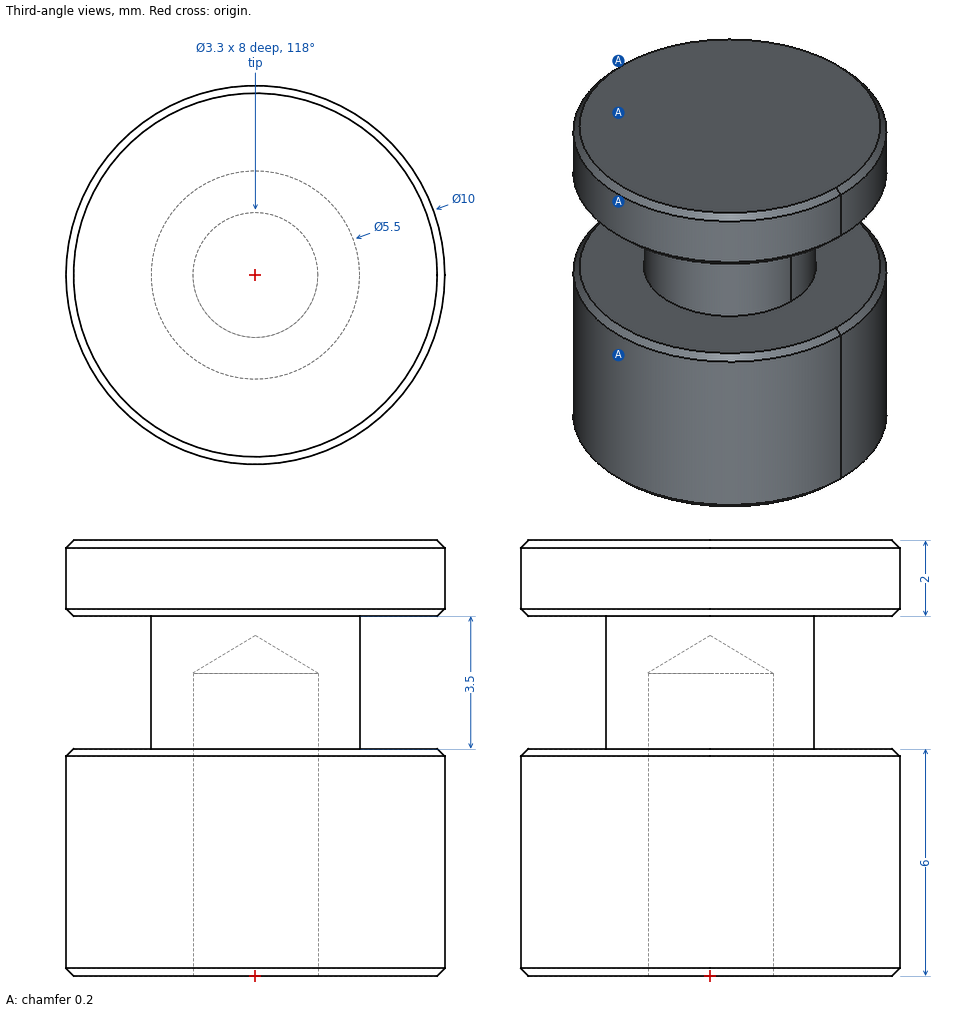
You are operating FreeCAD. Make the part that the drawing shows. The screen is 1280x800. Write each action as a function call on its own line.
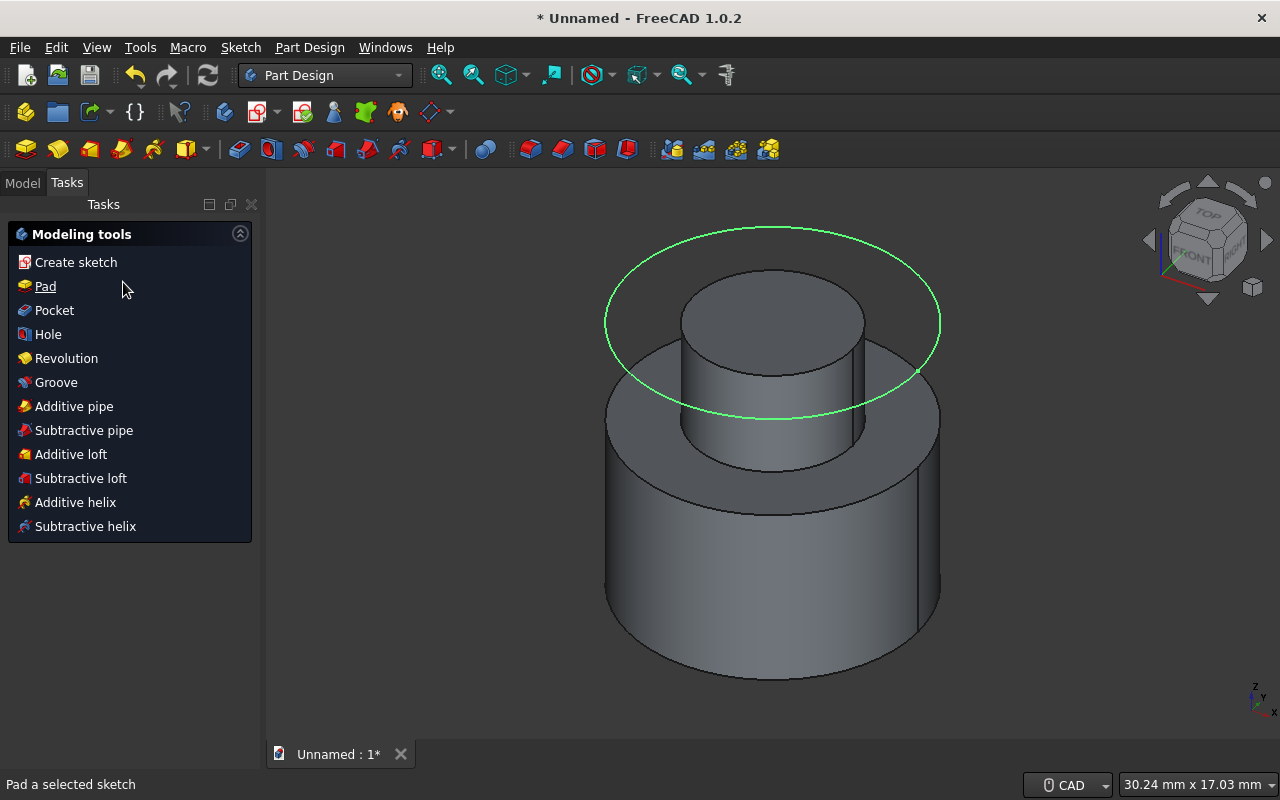
click(26, 150)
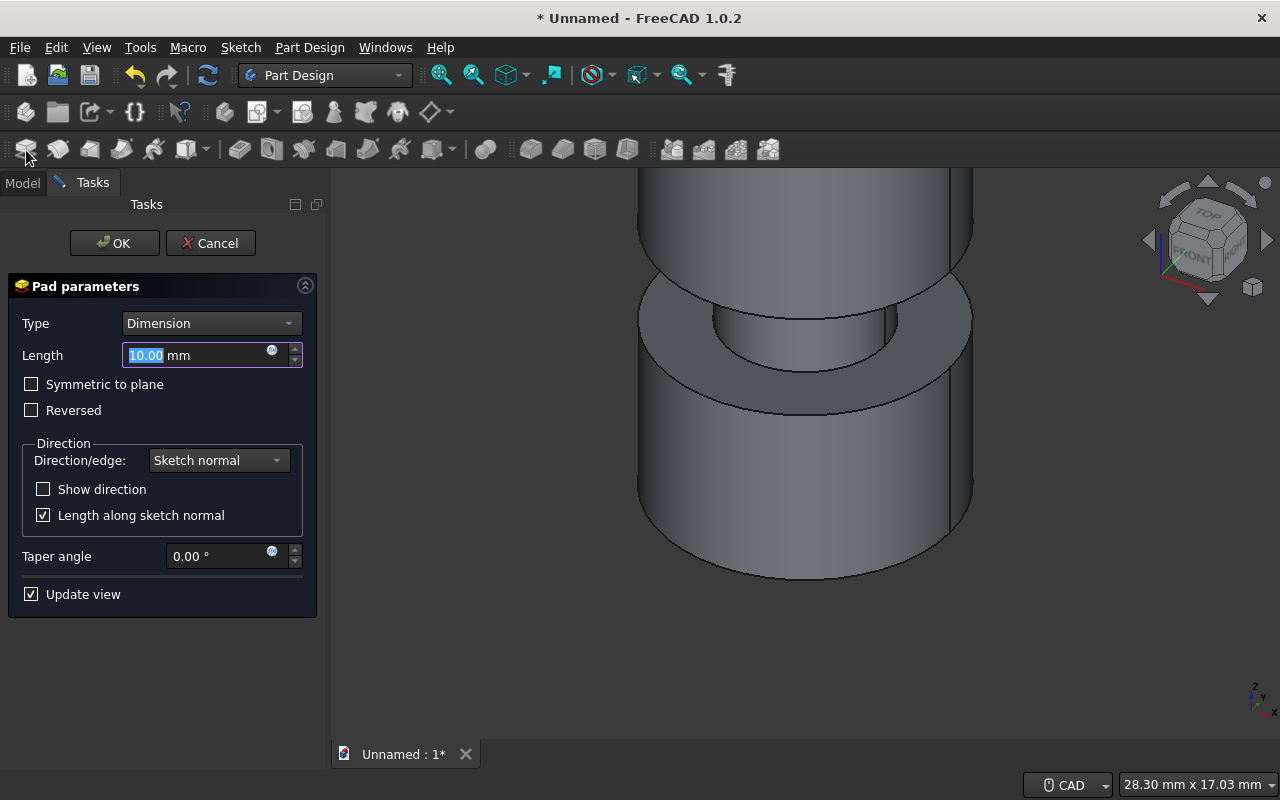
text(2)
key(Tab)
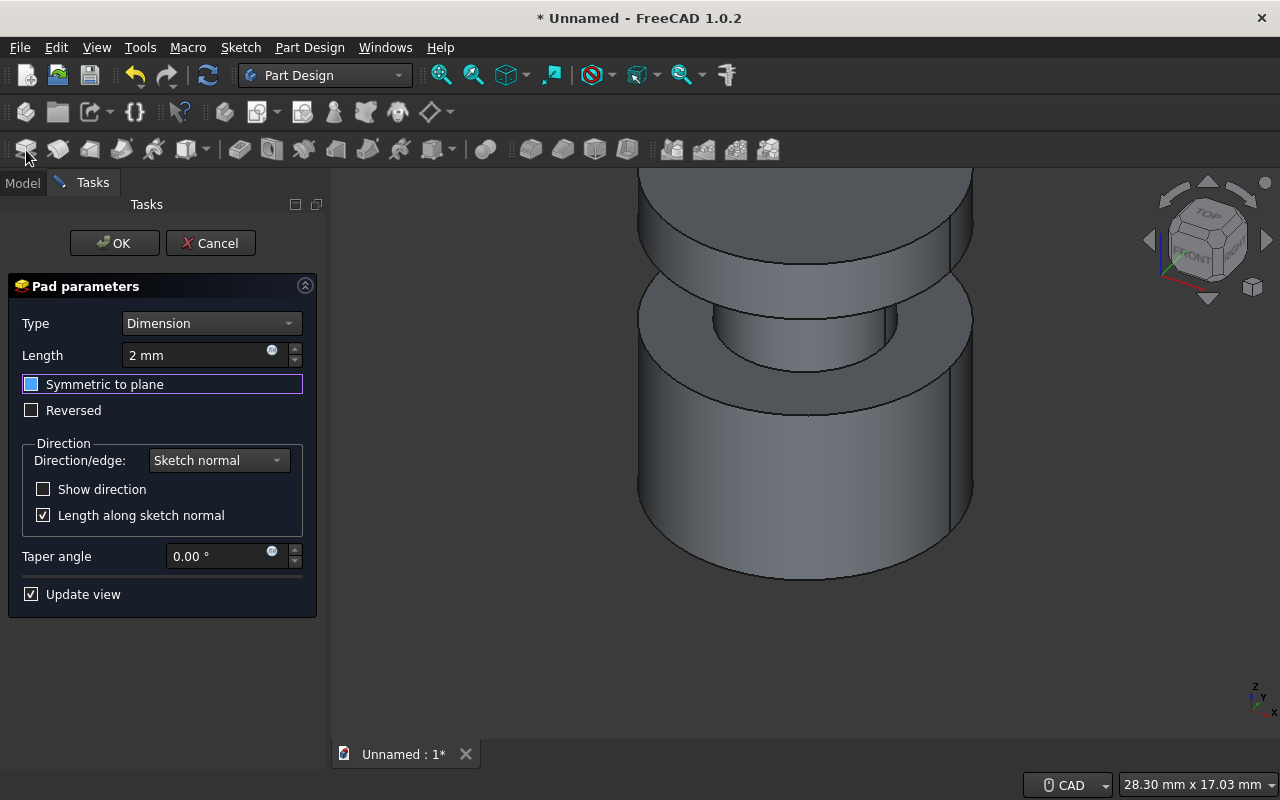
click(115, 243)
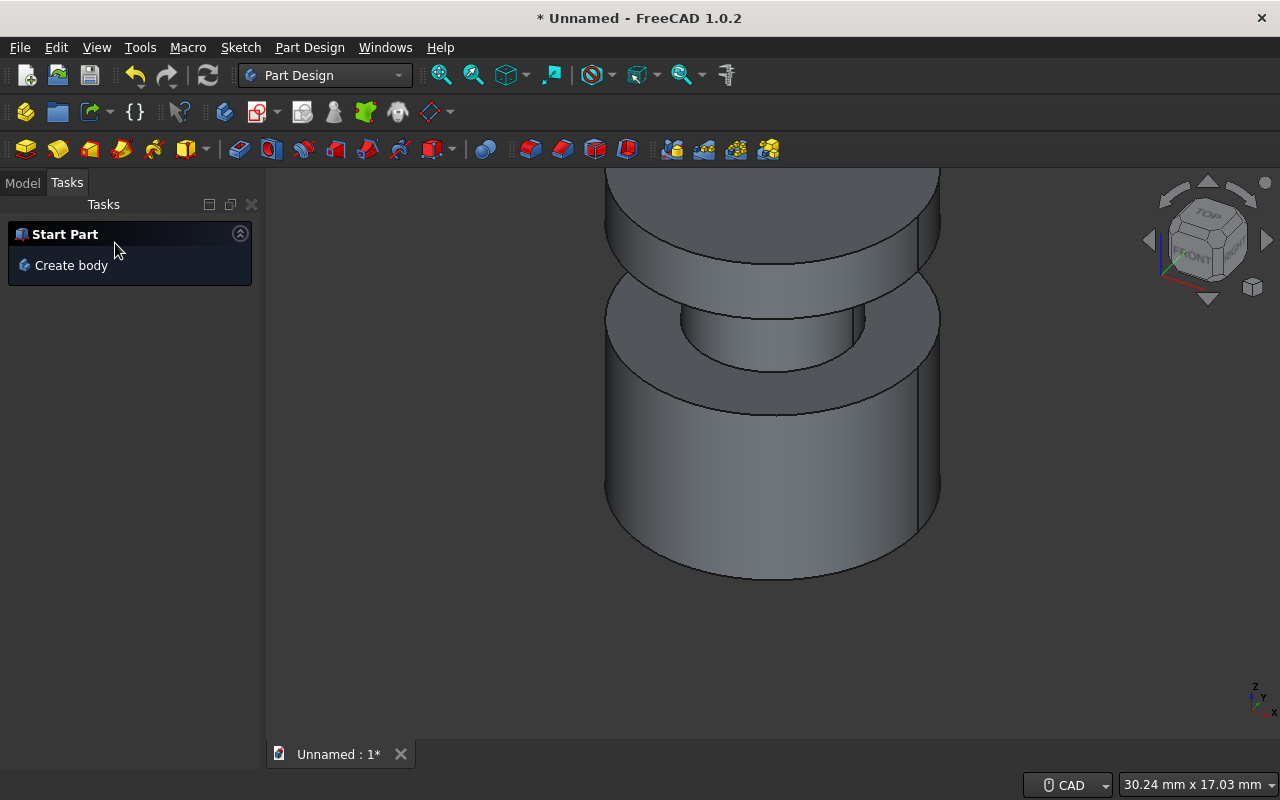
key(v)
key(f)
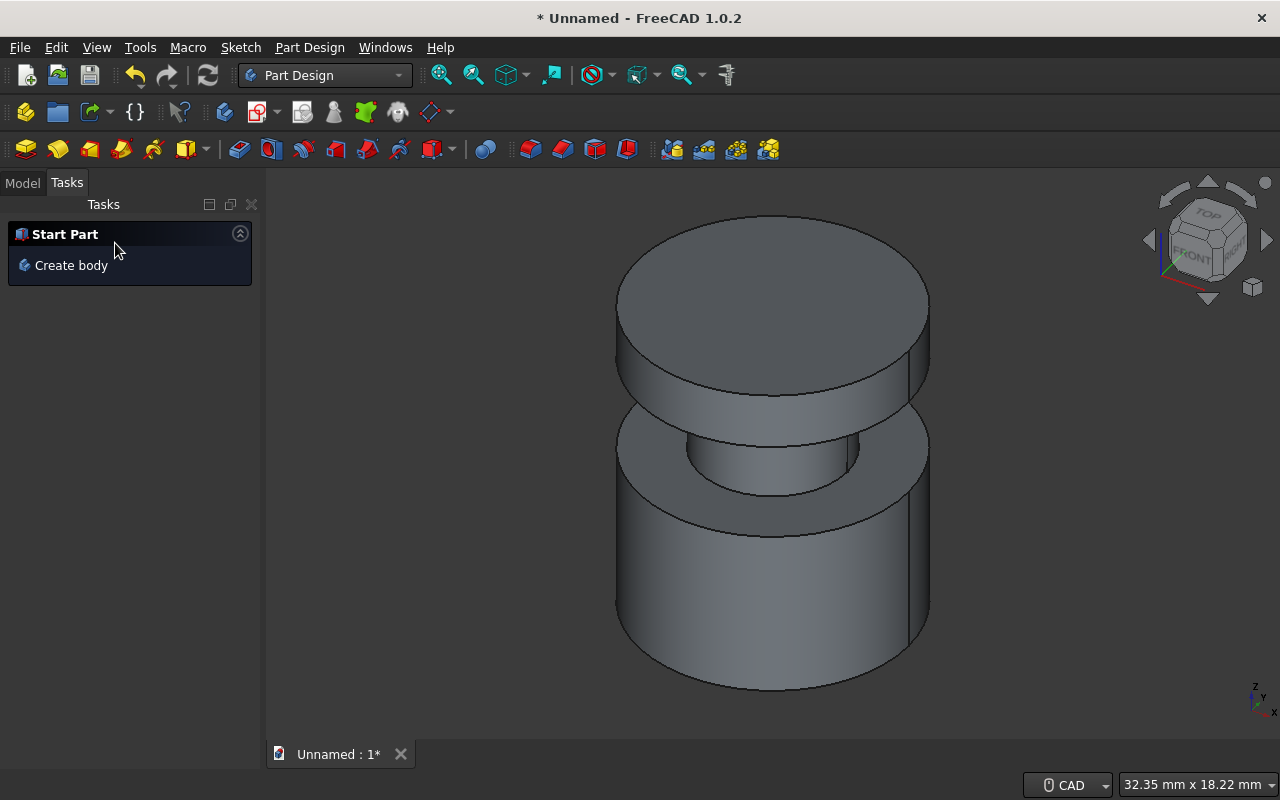
key(5)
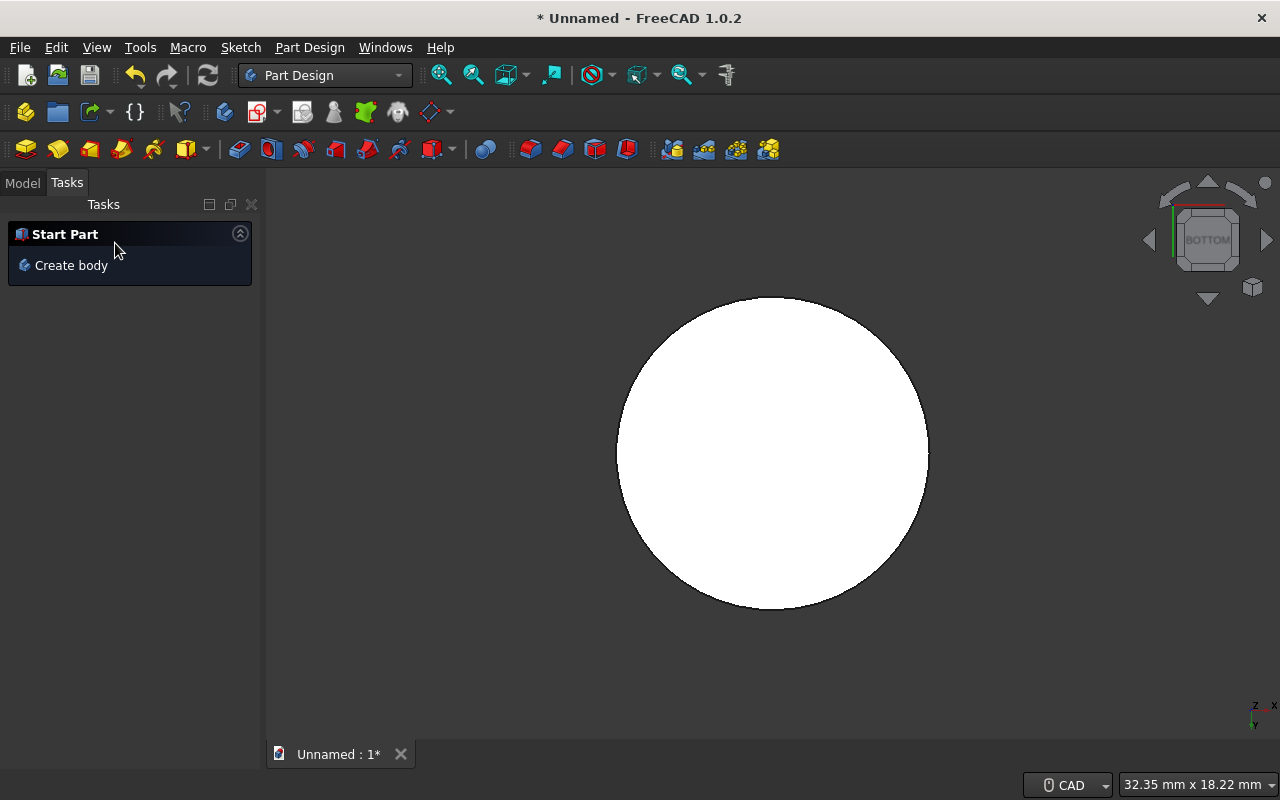
click(773, 452)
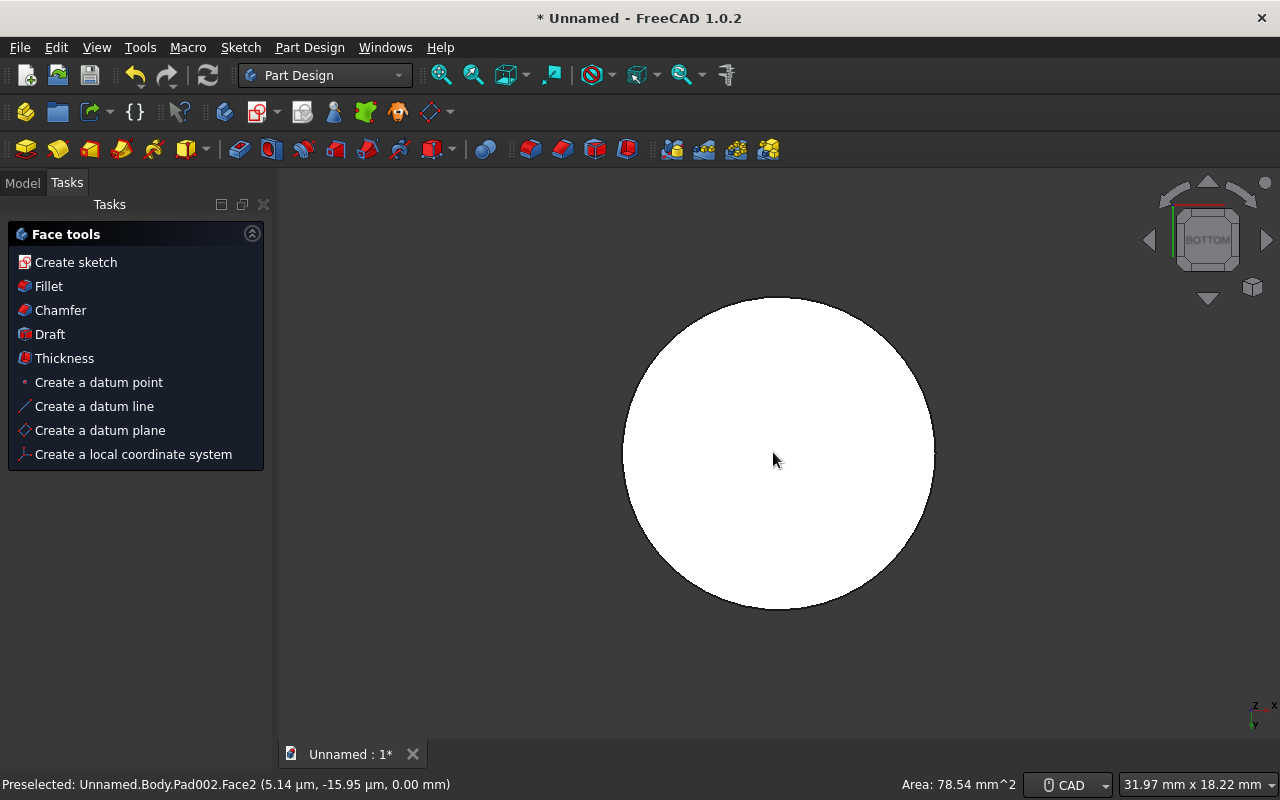
click(258, 112)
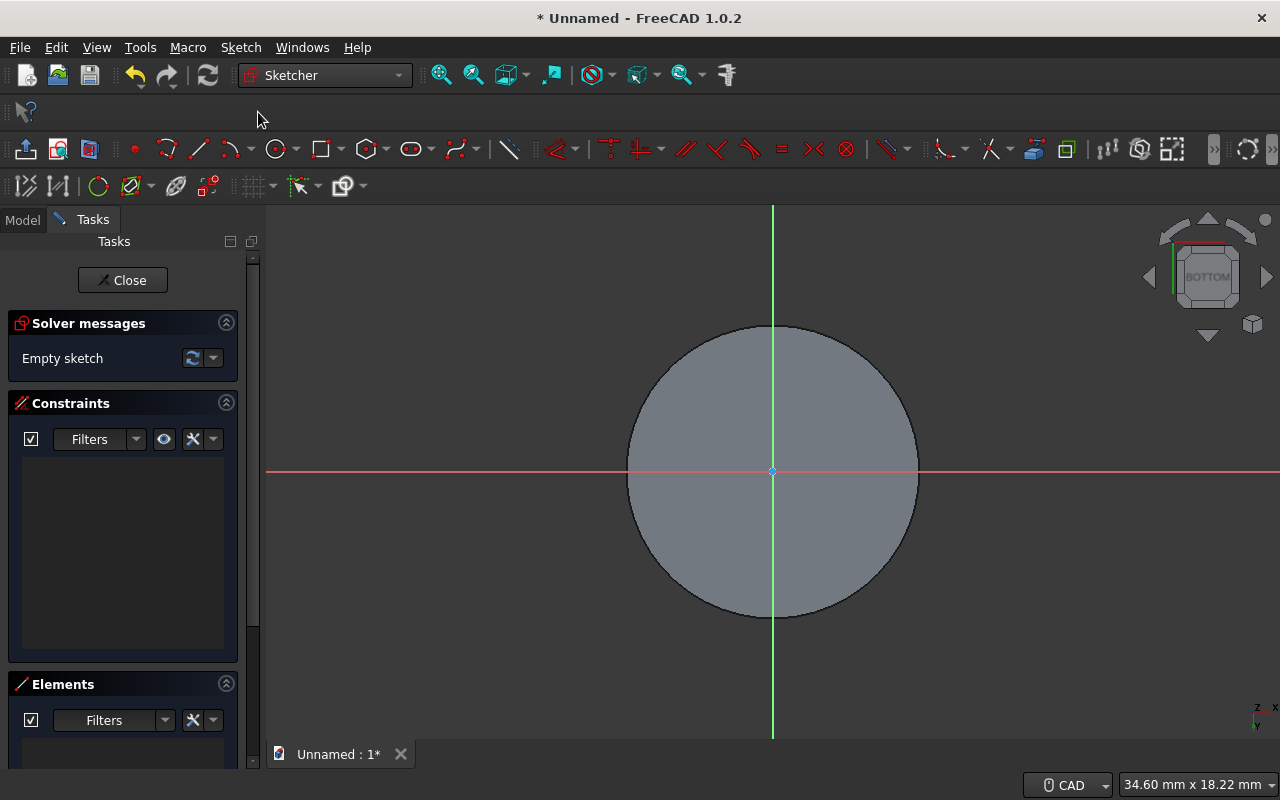
scroll(802, 472, up, 6)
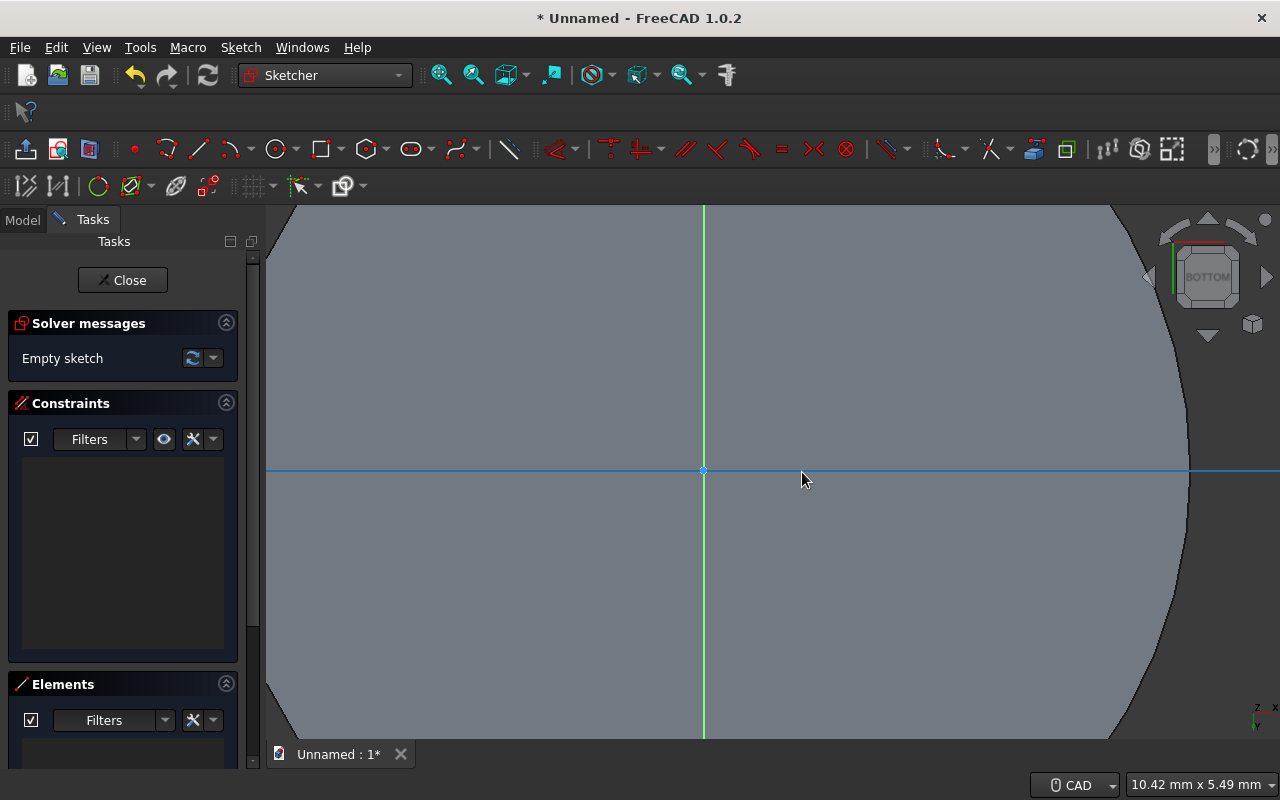
click(276, 150)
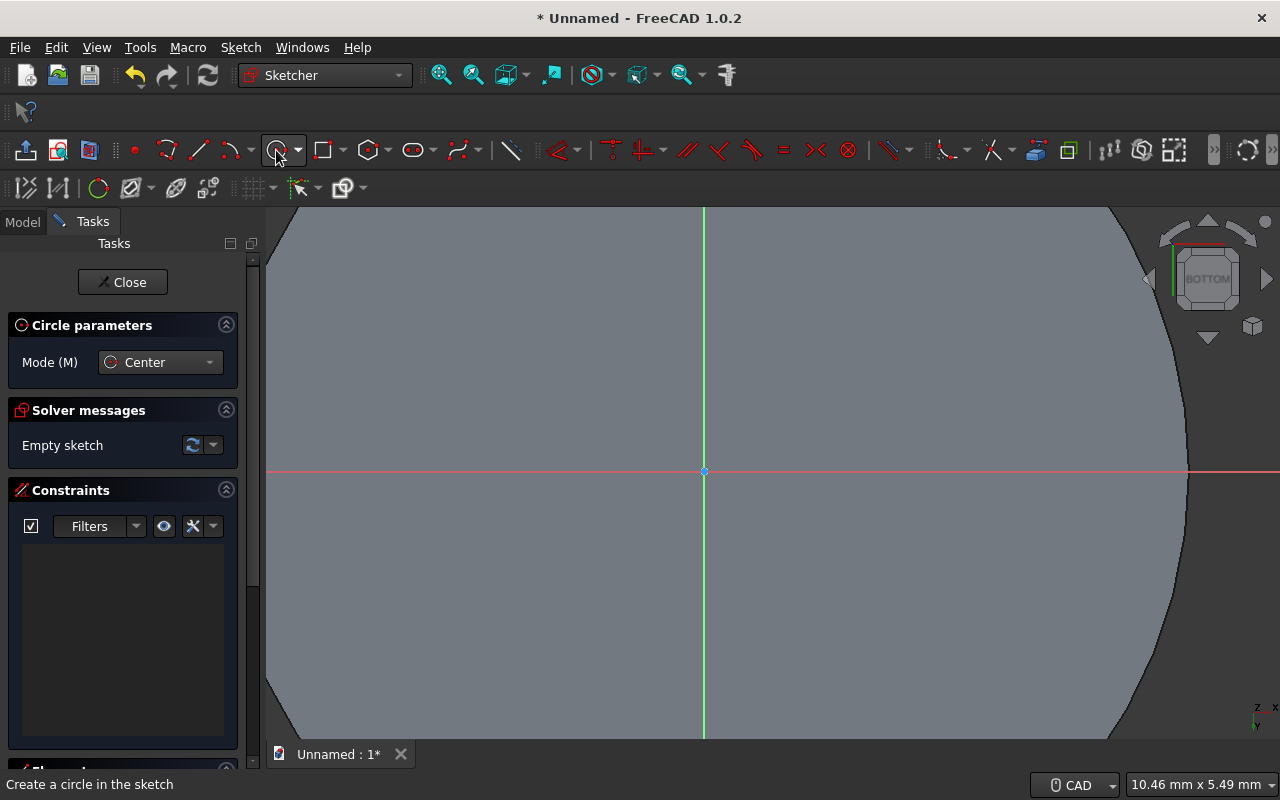
click(704, 472)
move(817, 359)